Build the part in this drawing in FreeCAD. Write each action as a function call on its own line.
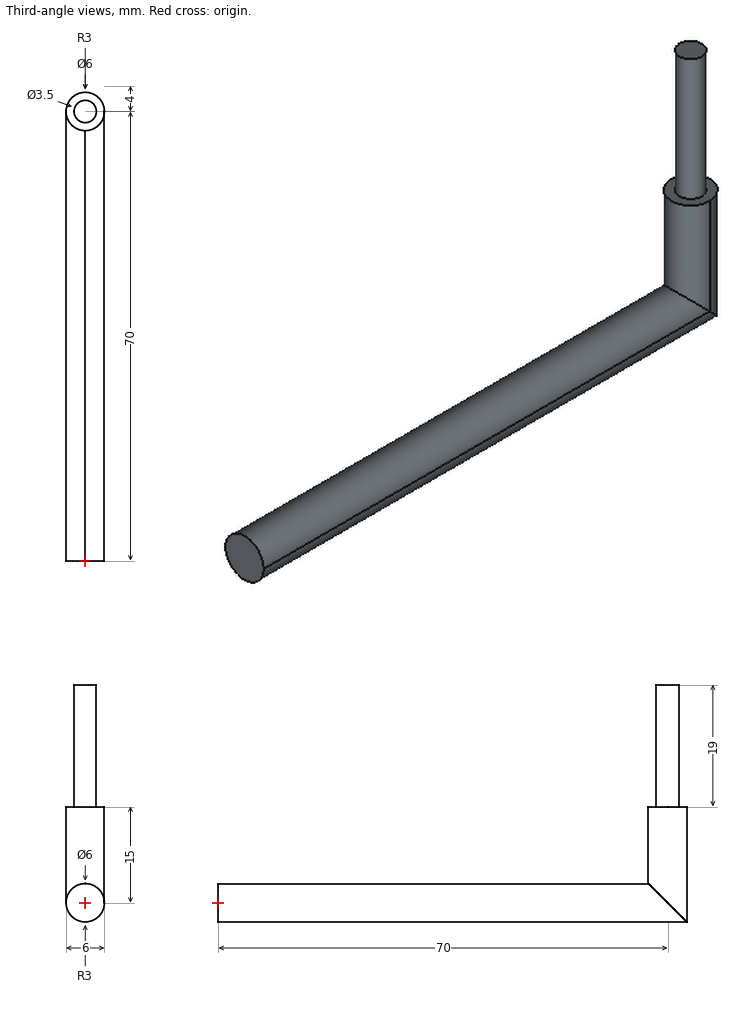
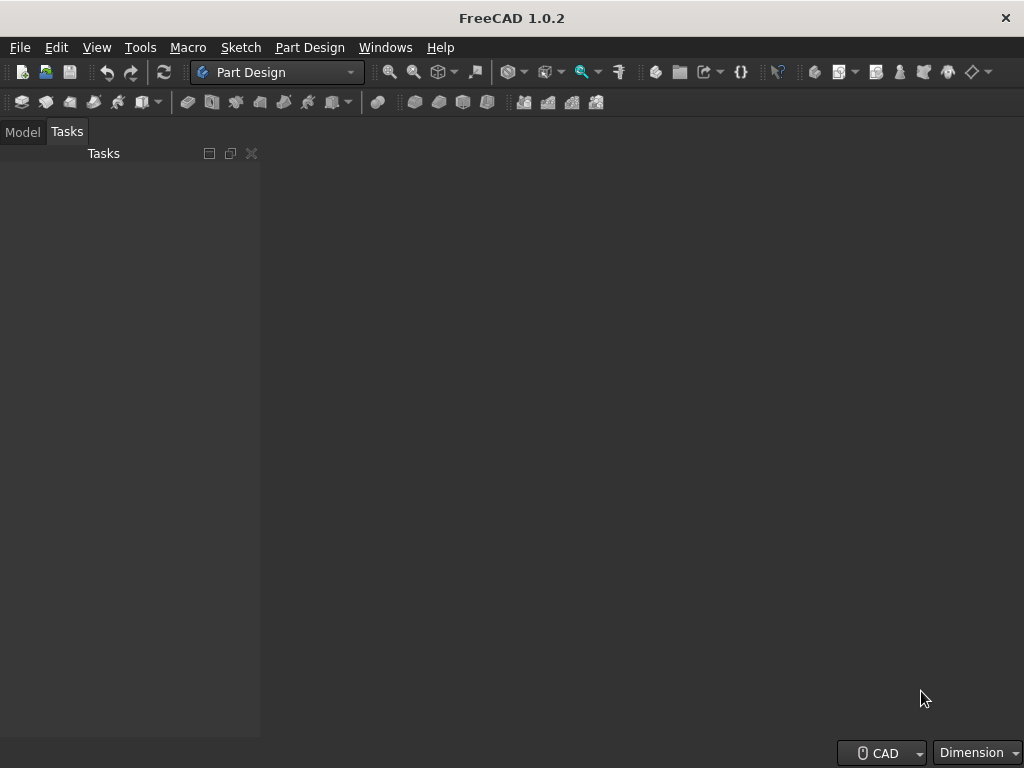
key(ctrl+n)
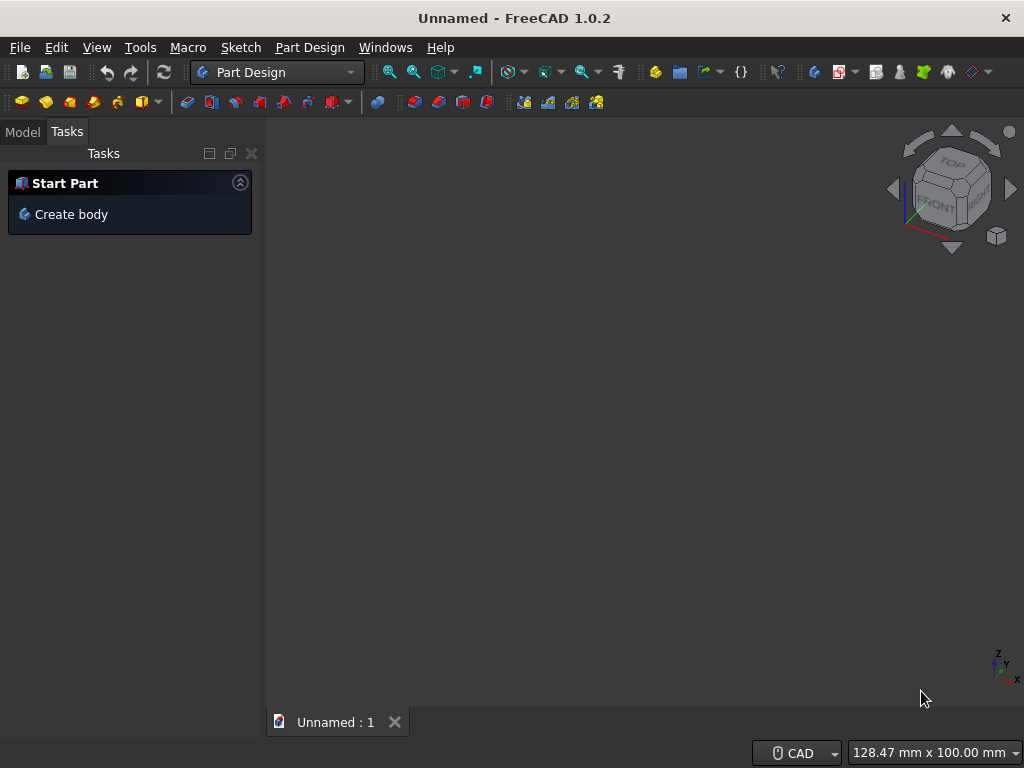
click(840, 72)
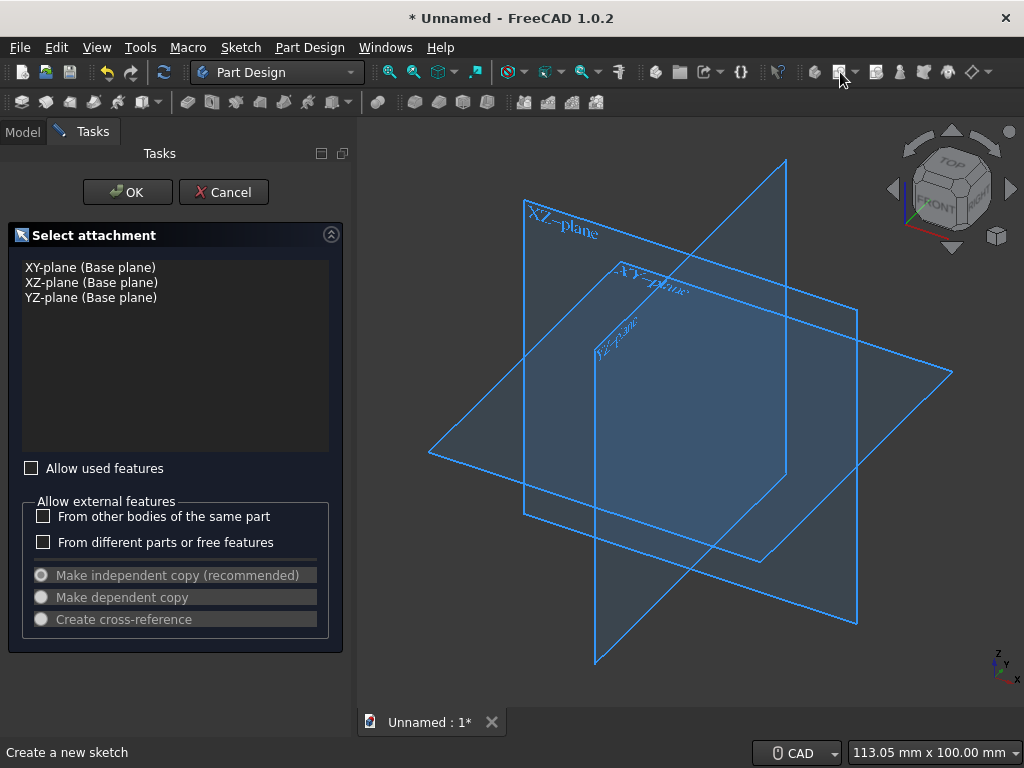
click(82, 282)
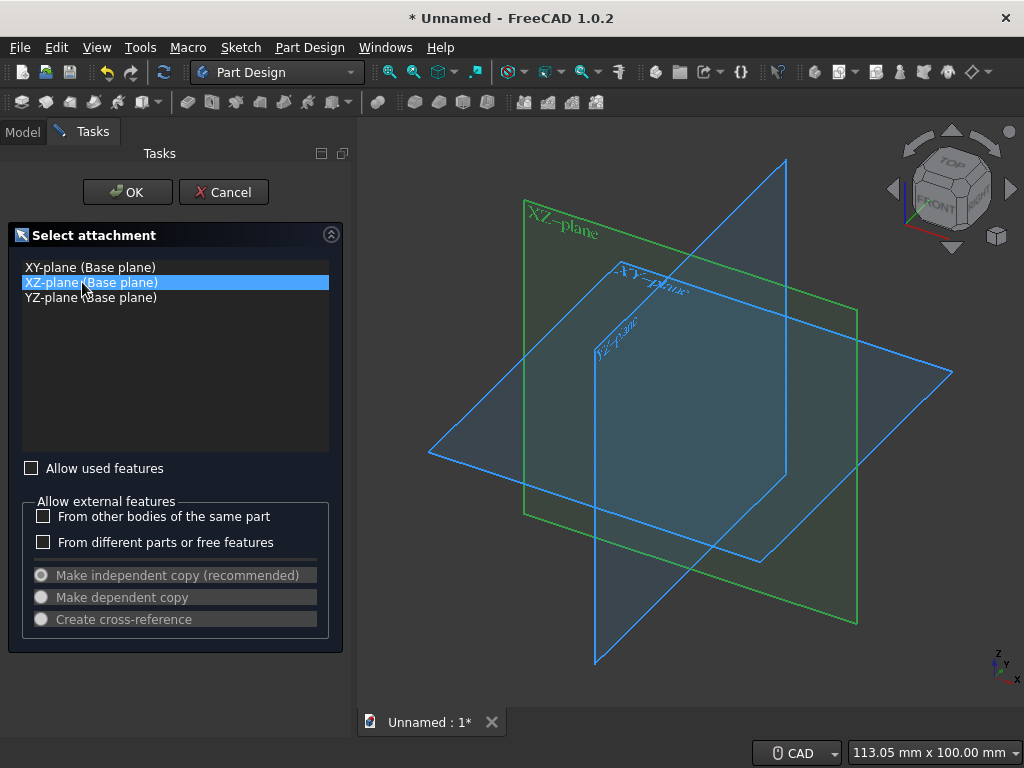
click(128, 192)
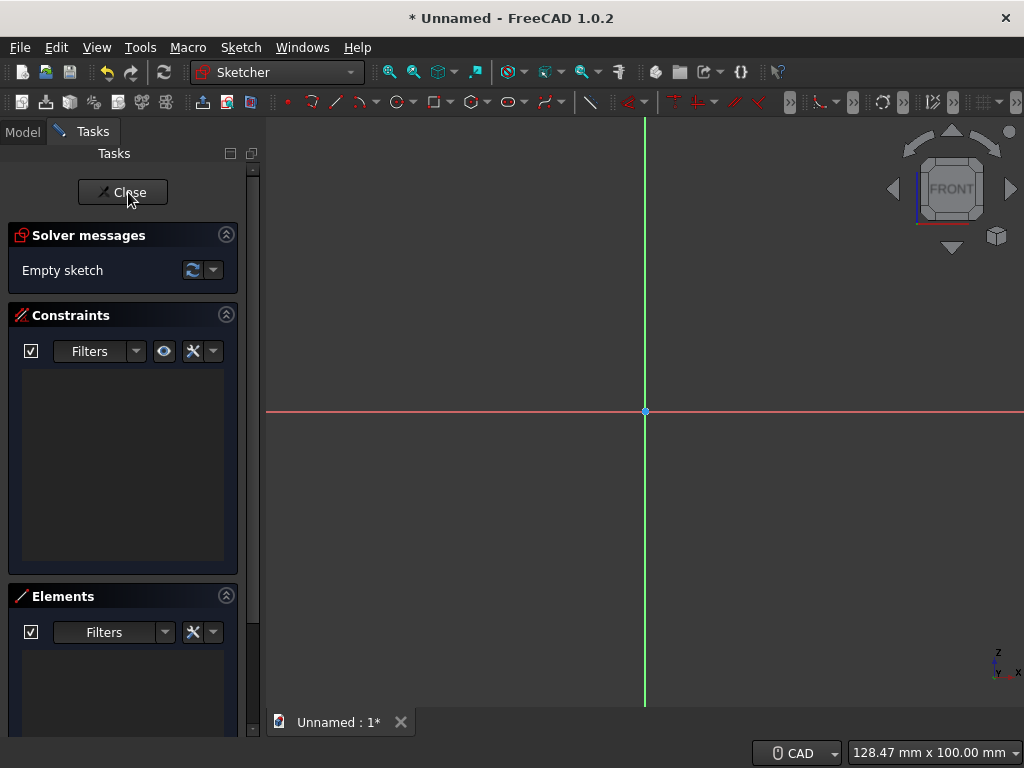
scroll(652, 412, up, 12)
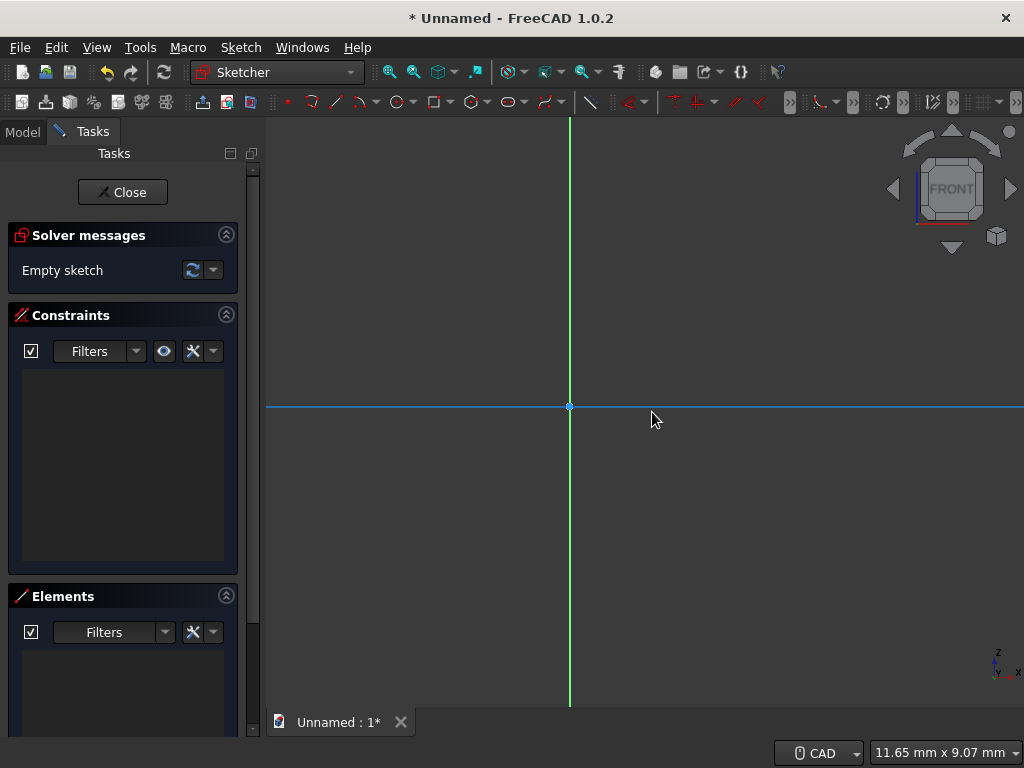
click(398, 102)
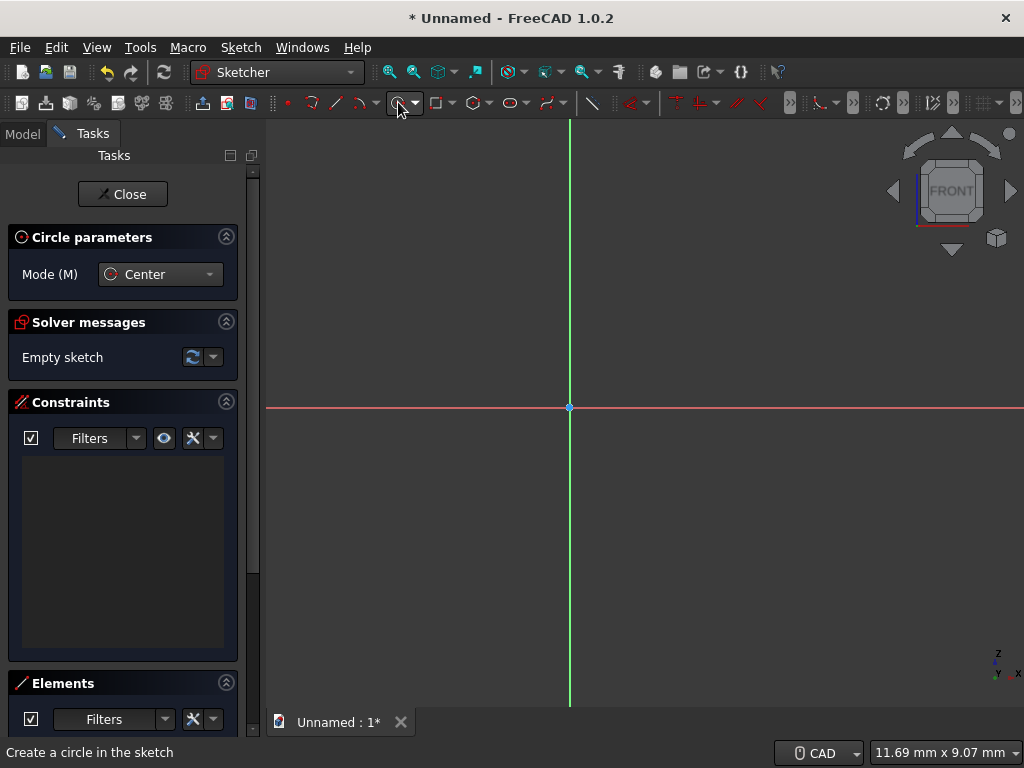
click(570, 408)
click(707, 271)
key(Escape)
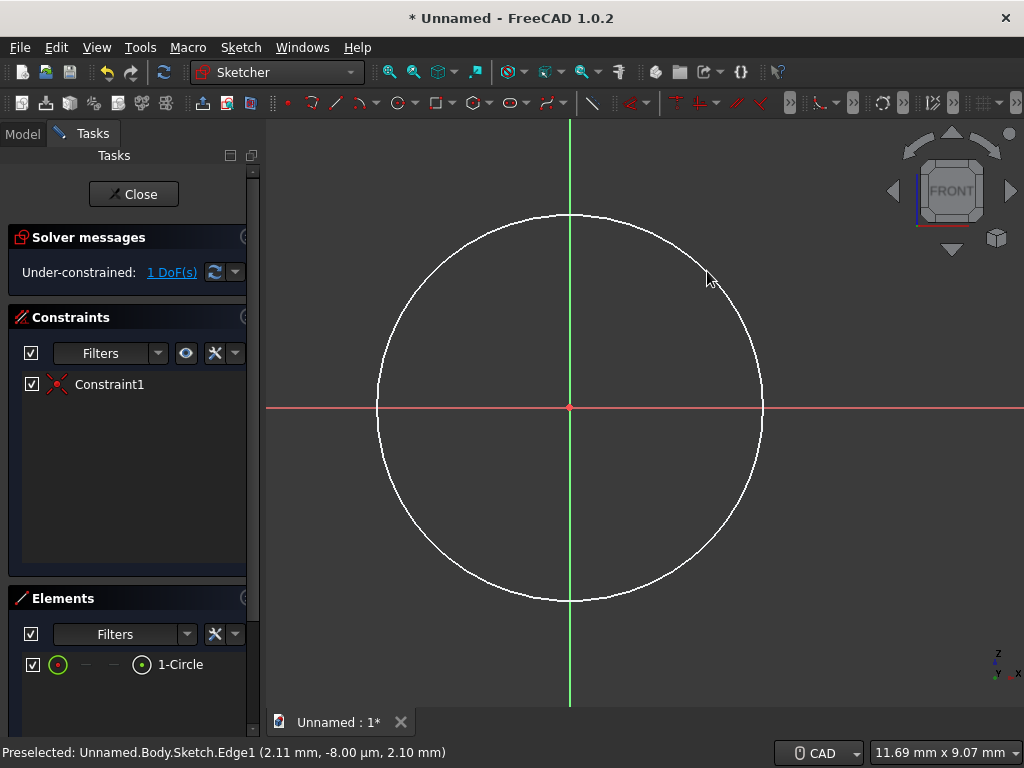
key(d)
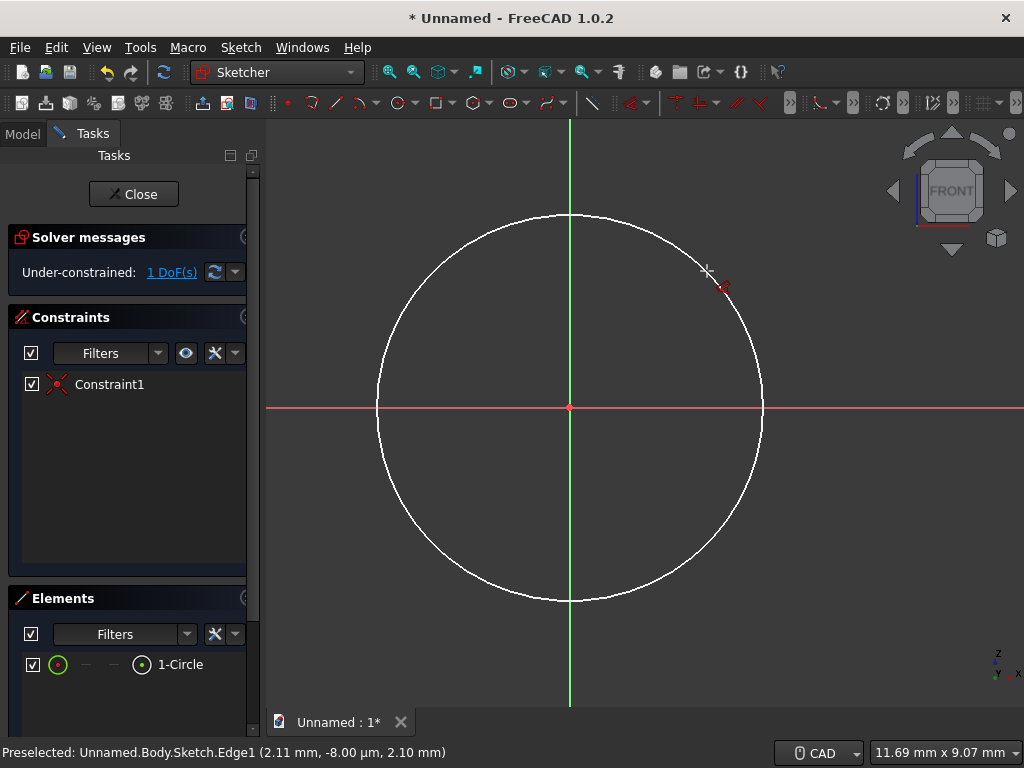
click(706, 271)
click(729, 248)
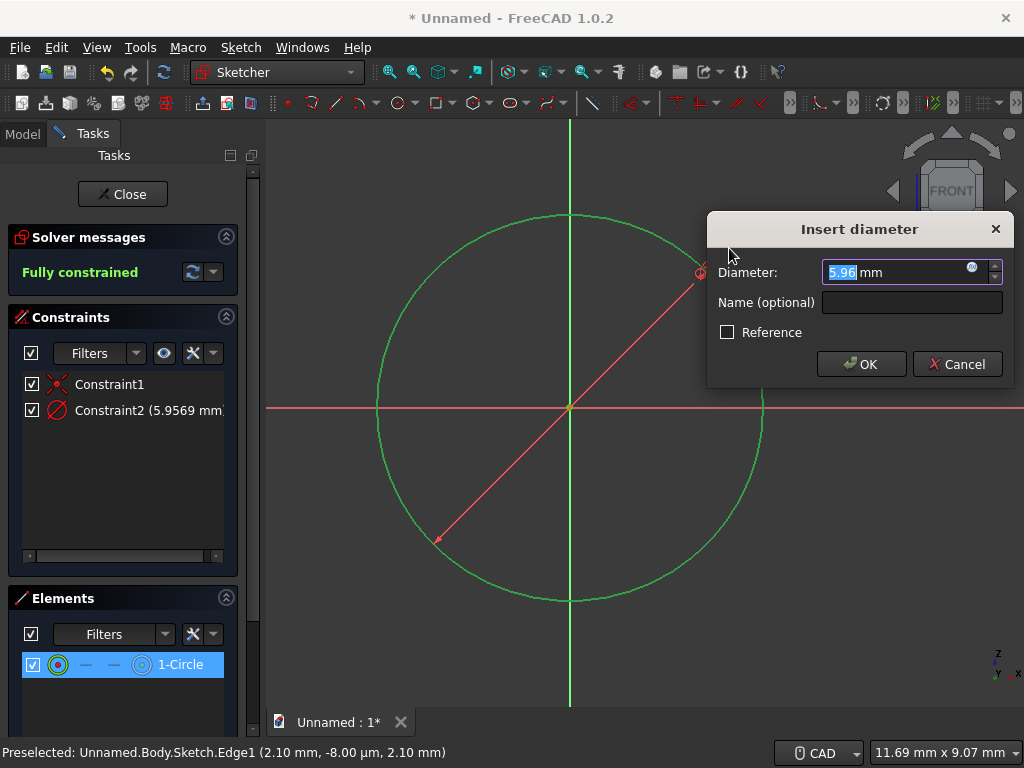
text(6)
key(Return)
key(Escape)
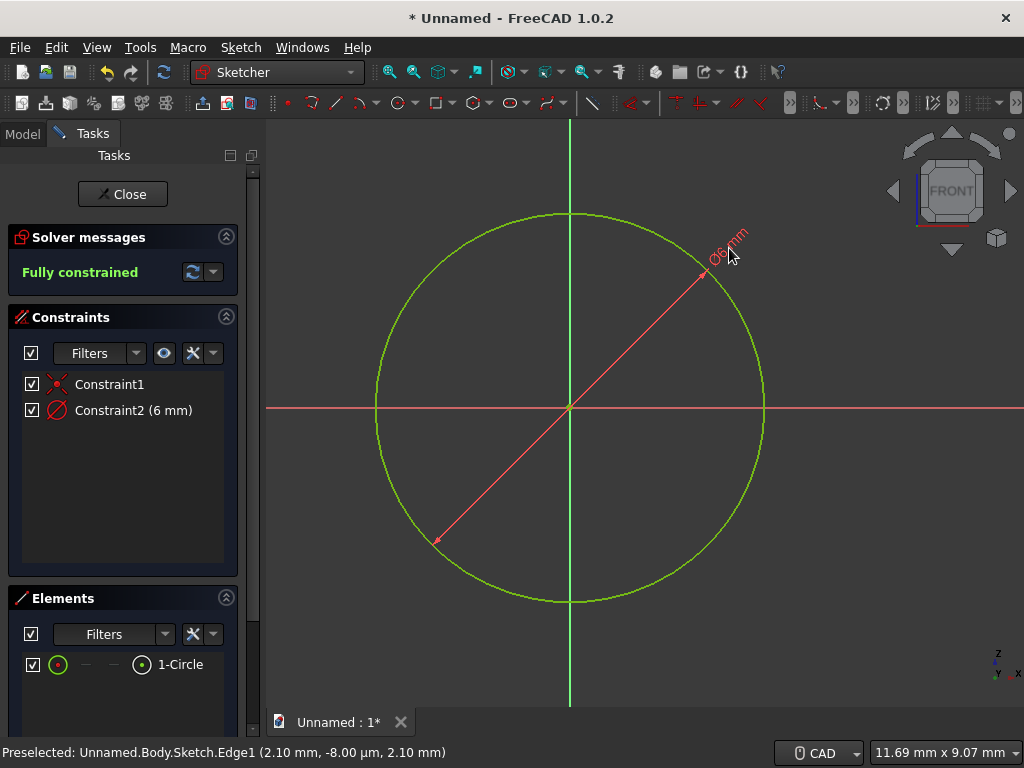
click(123, 194)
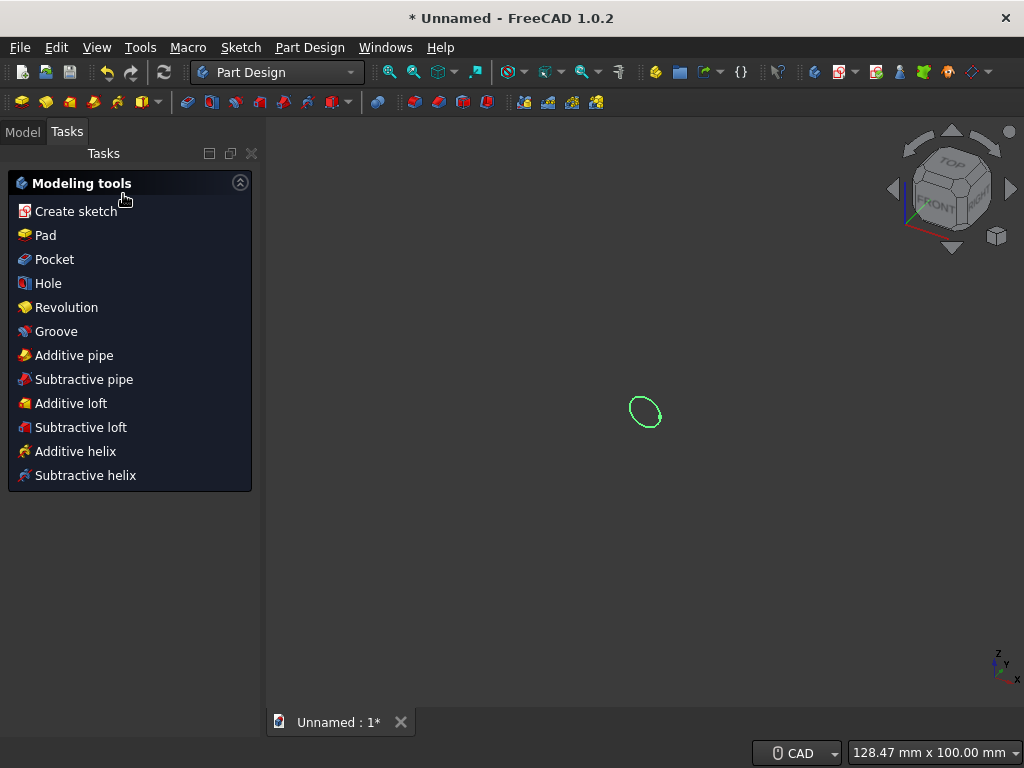
click(22, 102)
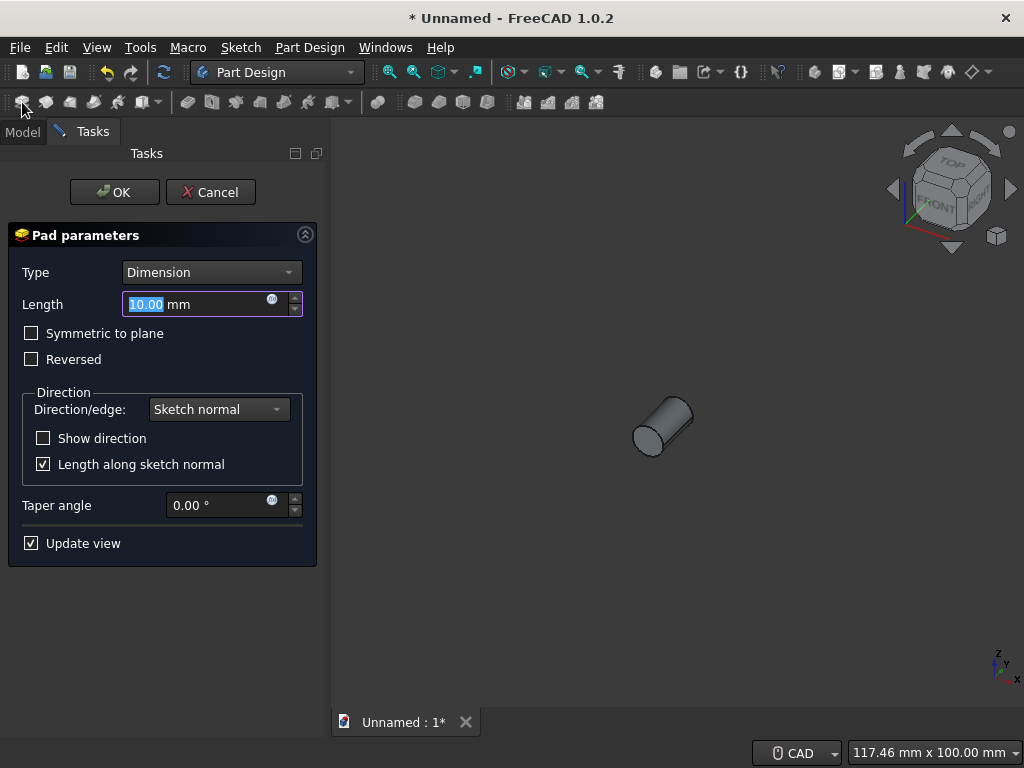
text(70)
key(Tab)